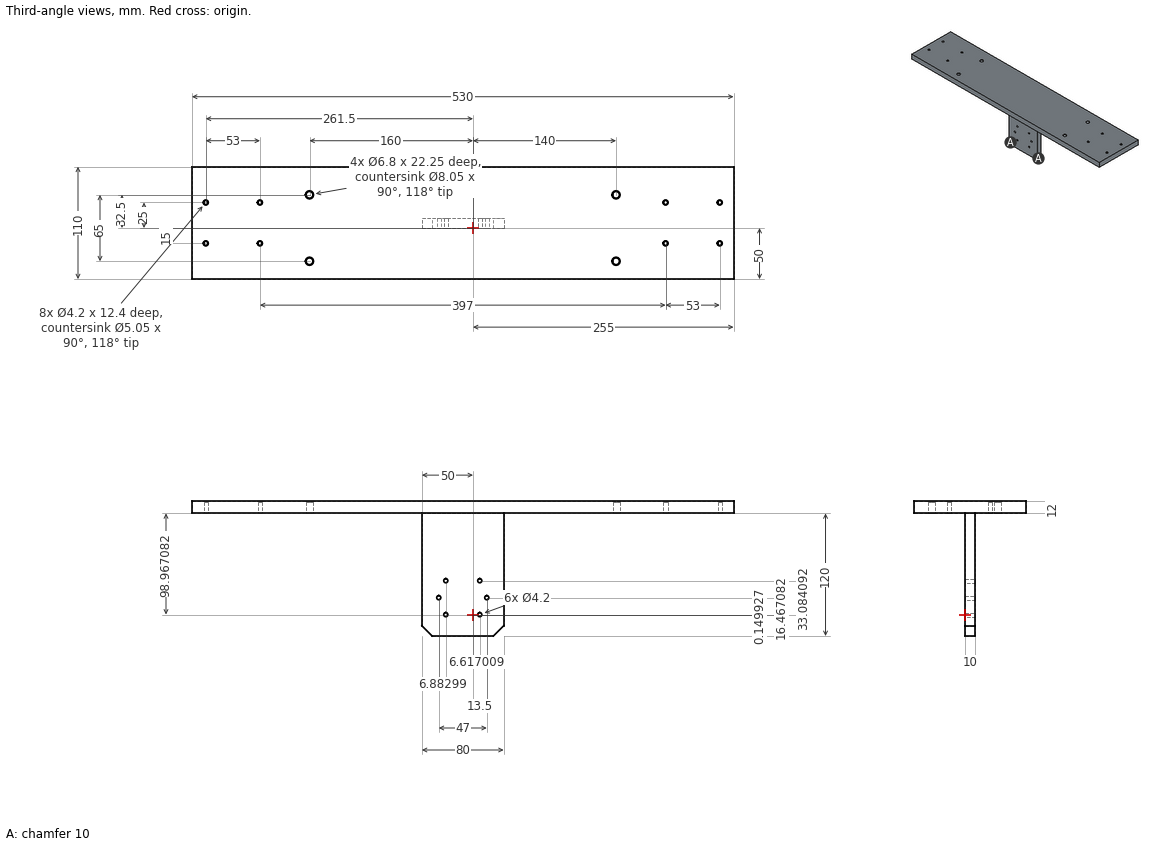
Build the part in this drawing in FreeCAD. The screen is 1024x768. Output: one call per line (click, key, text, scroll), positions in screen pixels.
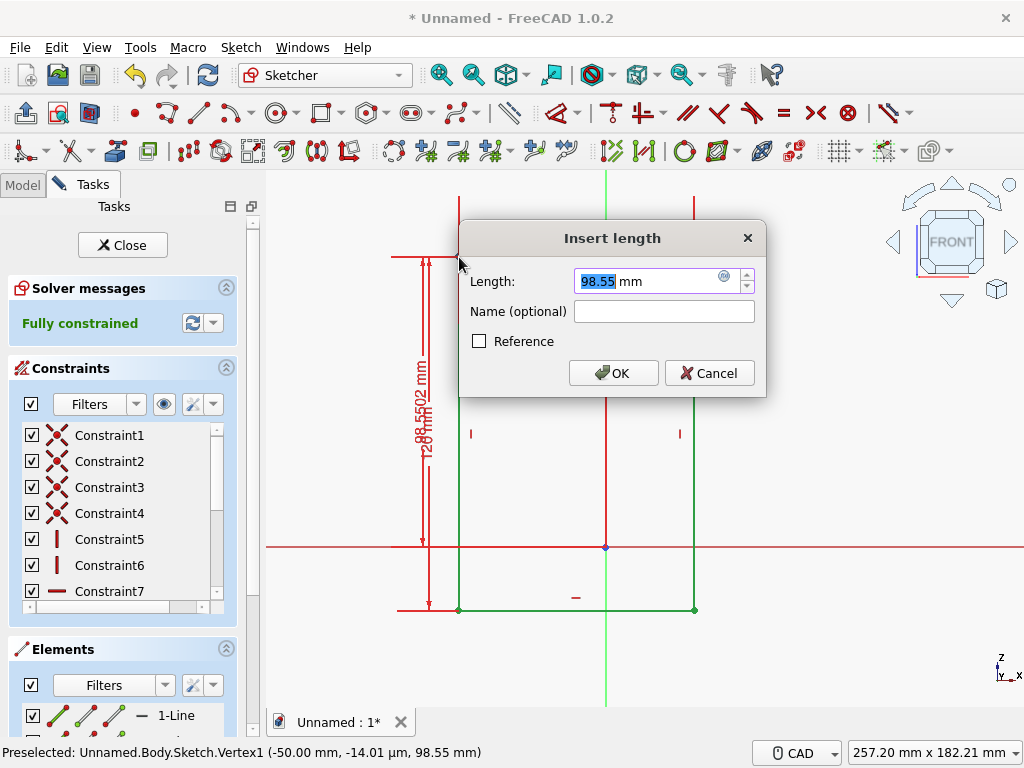
text(98.967082)
key(Return)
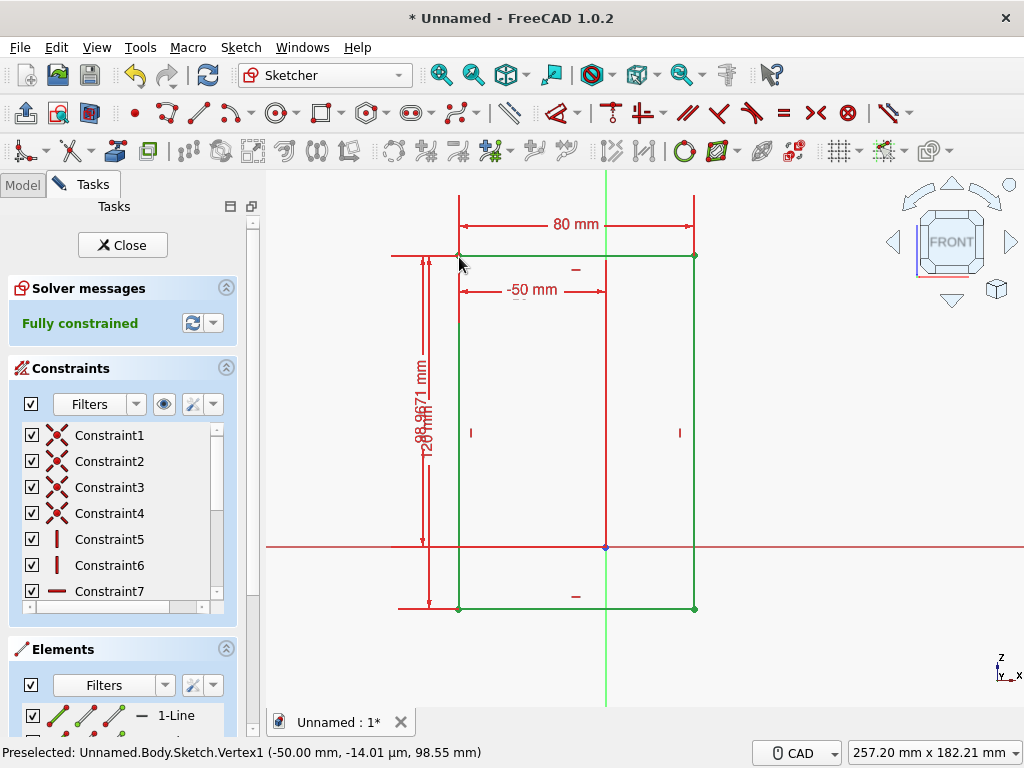
click(123, 245)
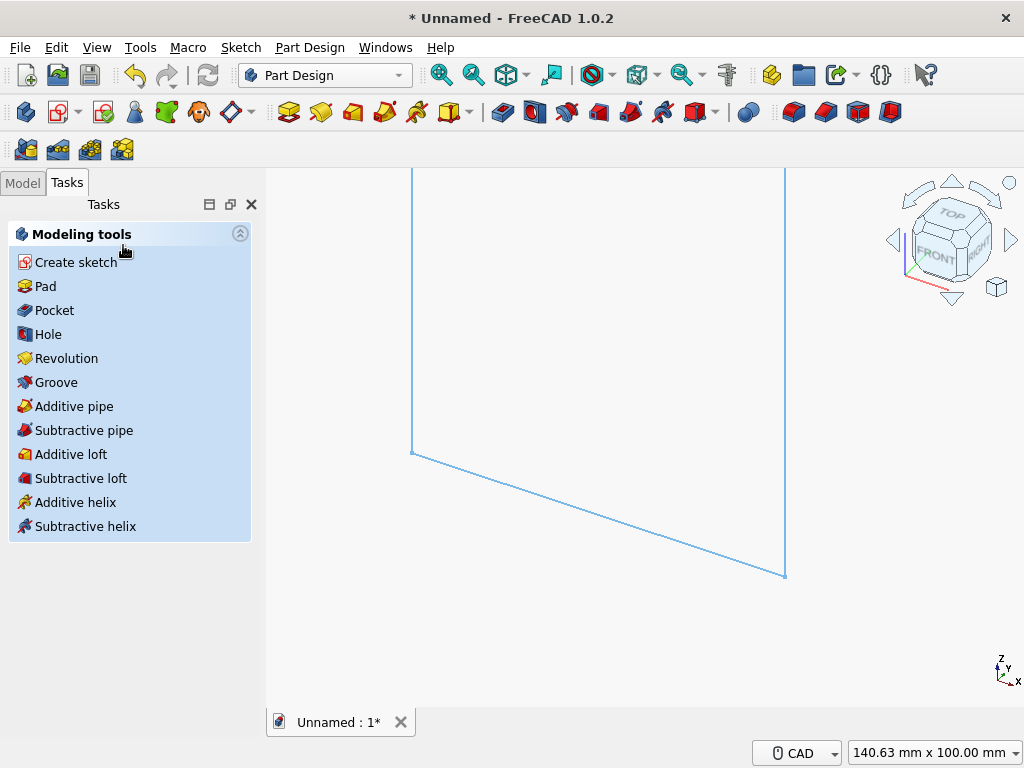
click(290, 112)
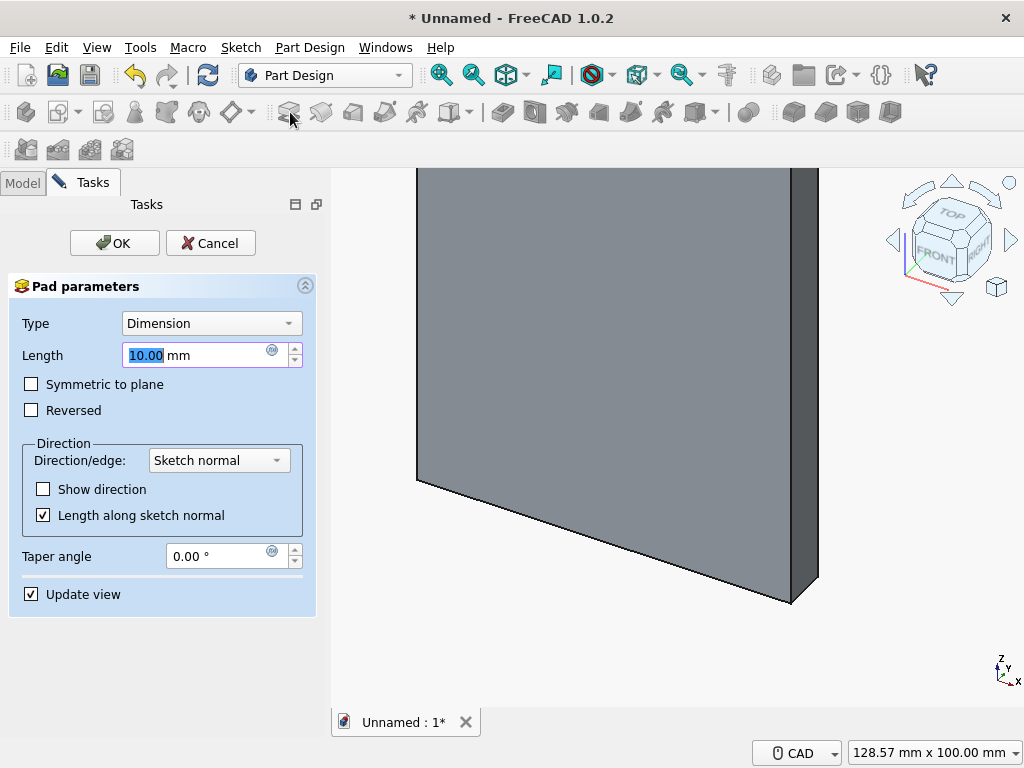
text(10)
key(Tab)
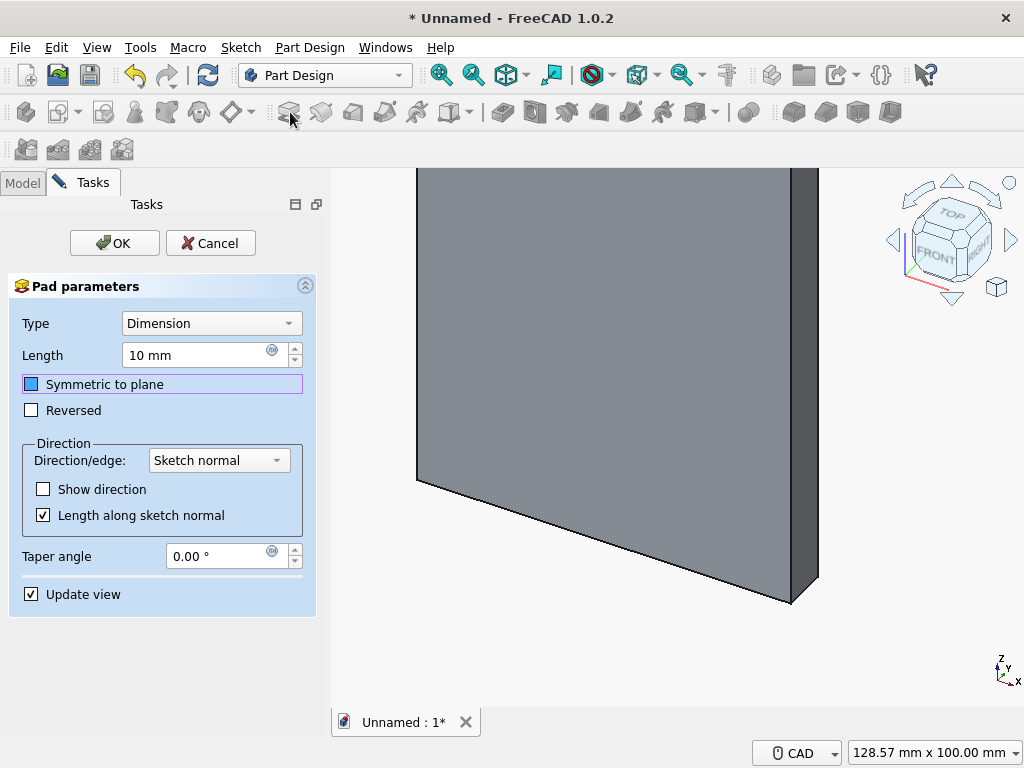
click(30, 410)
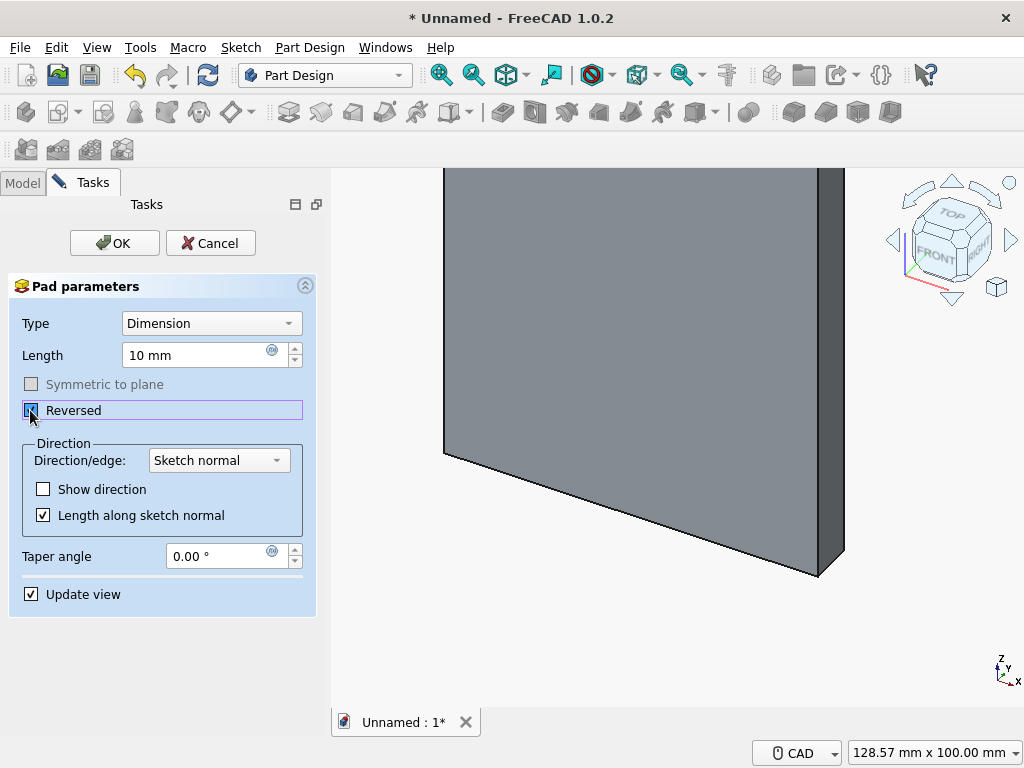
click(115, 243)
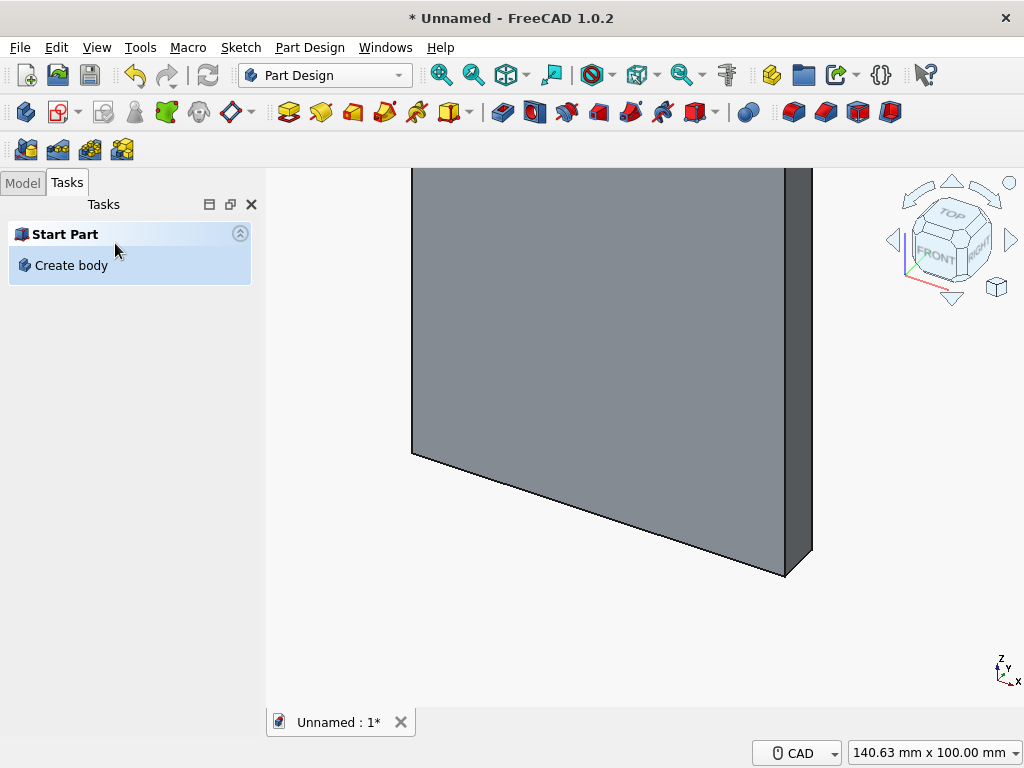
key(v)
key(f)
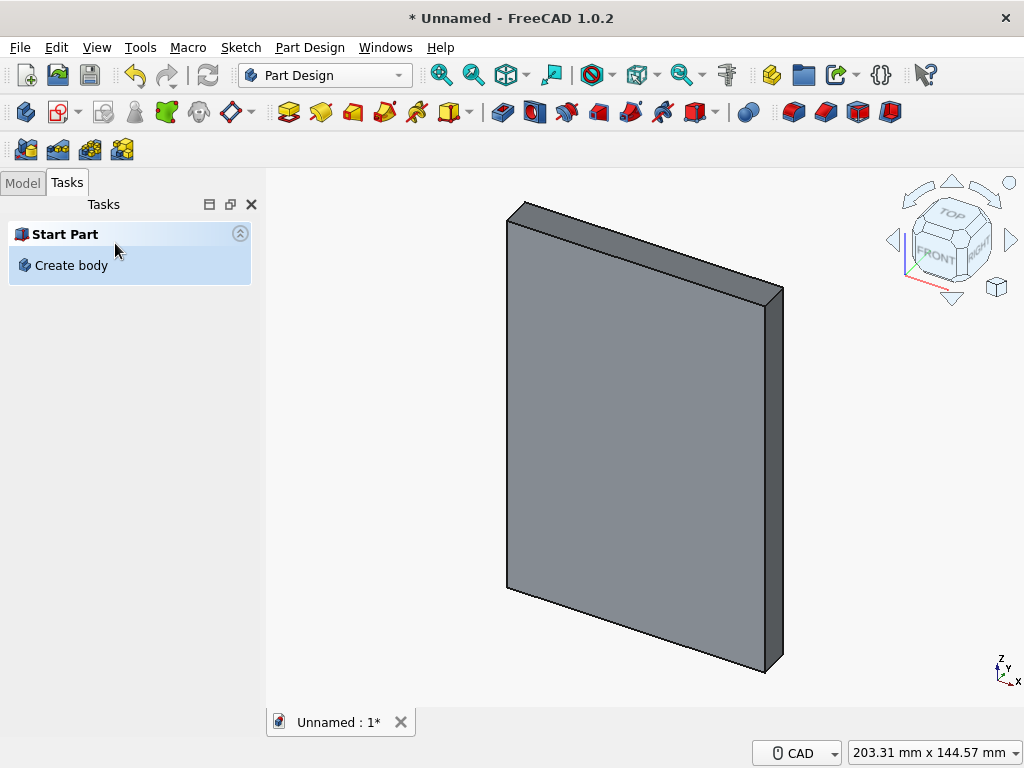
click(756, 290)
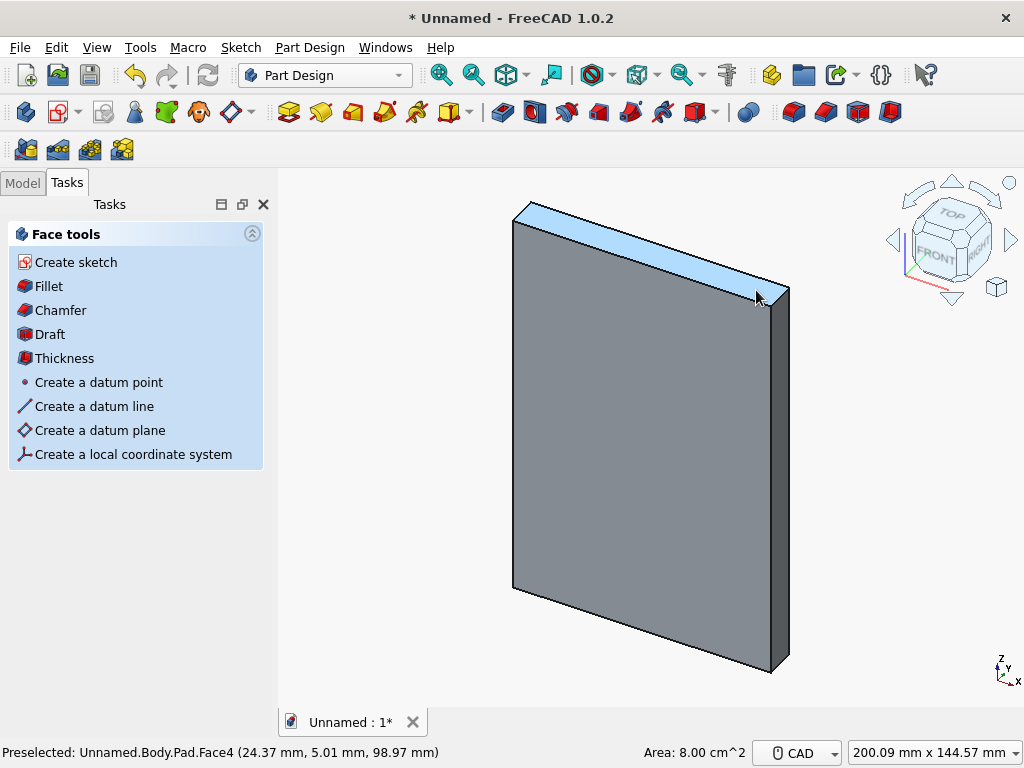
click(58, 112)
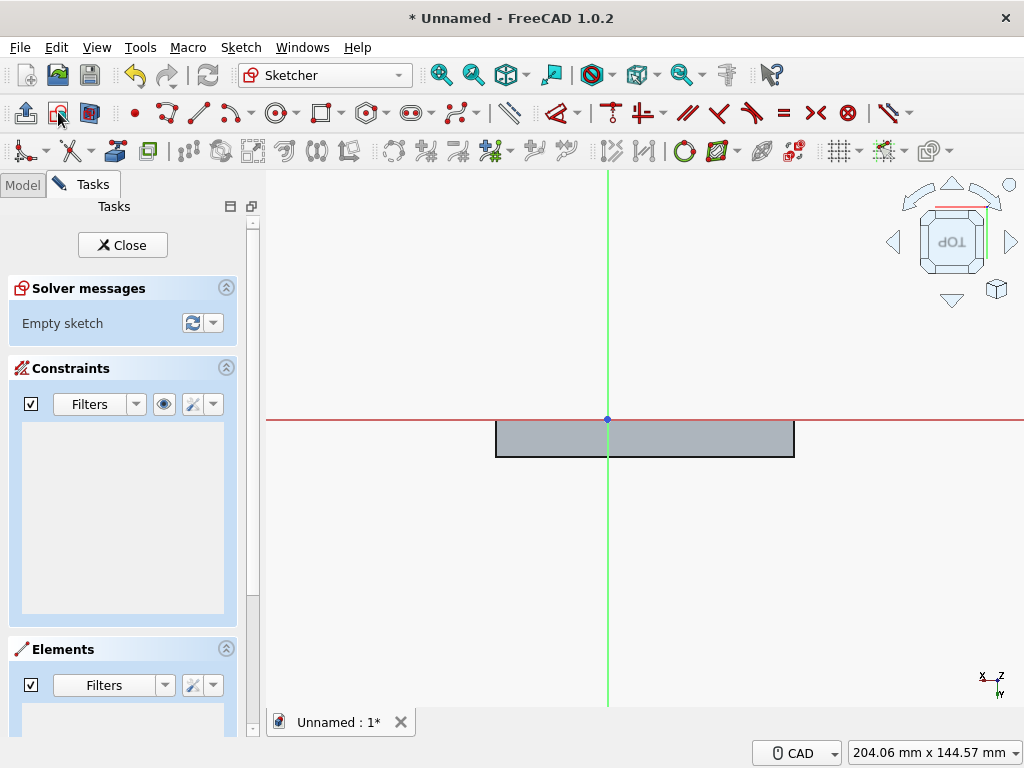
scroll(559, 438, down, 8)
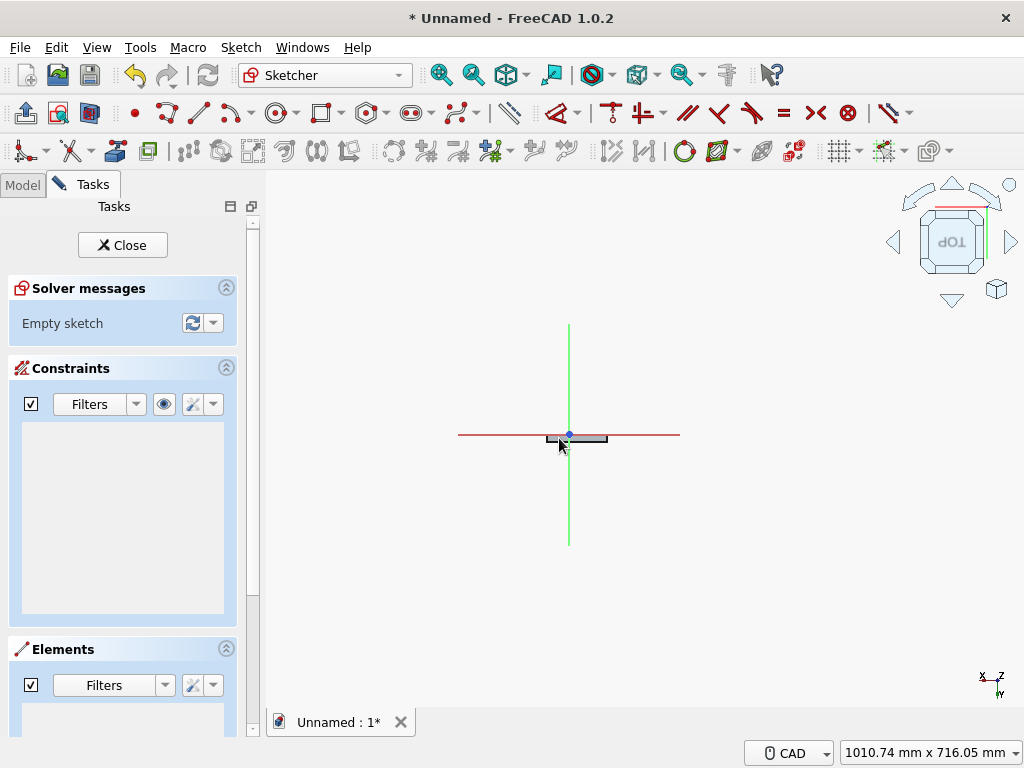
key(g)
key(r)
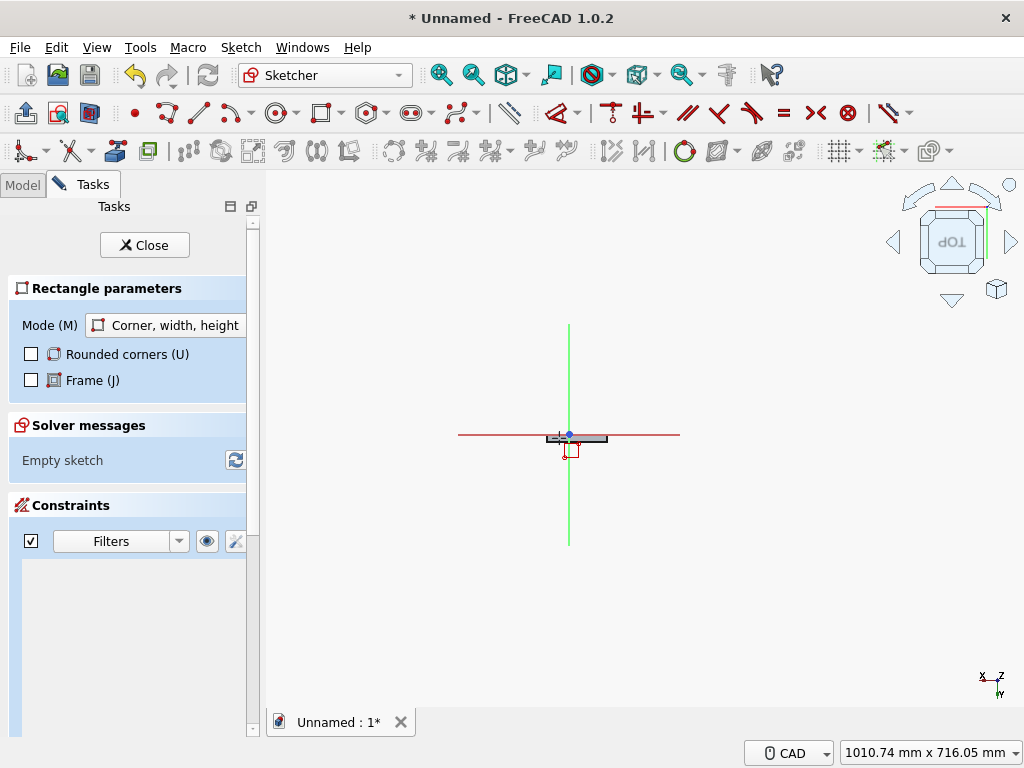
click(378, 397)
move(775, 480)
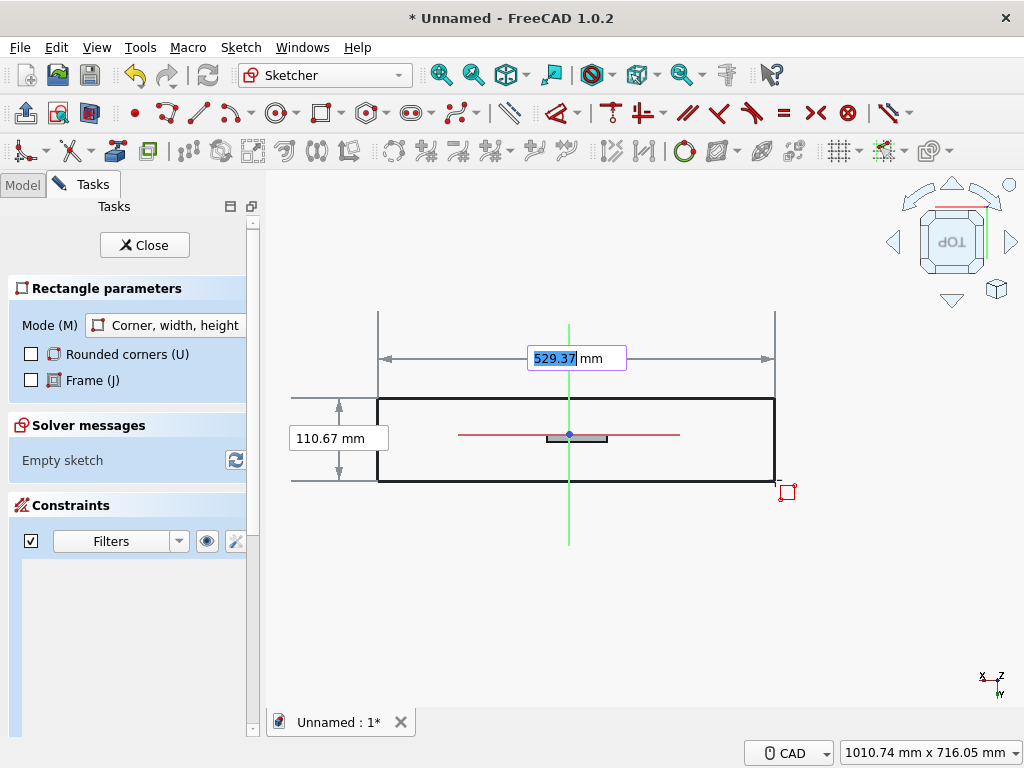
text(530)
key(Tab)
text(110)
key(Return)
key(Escape)